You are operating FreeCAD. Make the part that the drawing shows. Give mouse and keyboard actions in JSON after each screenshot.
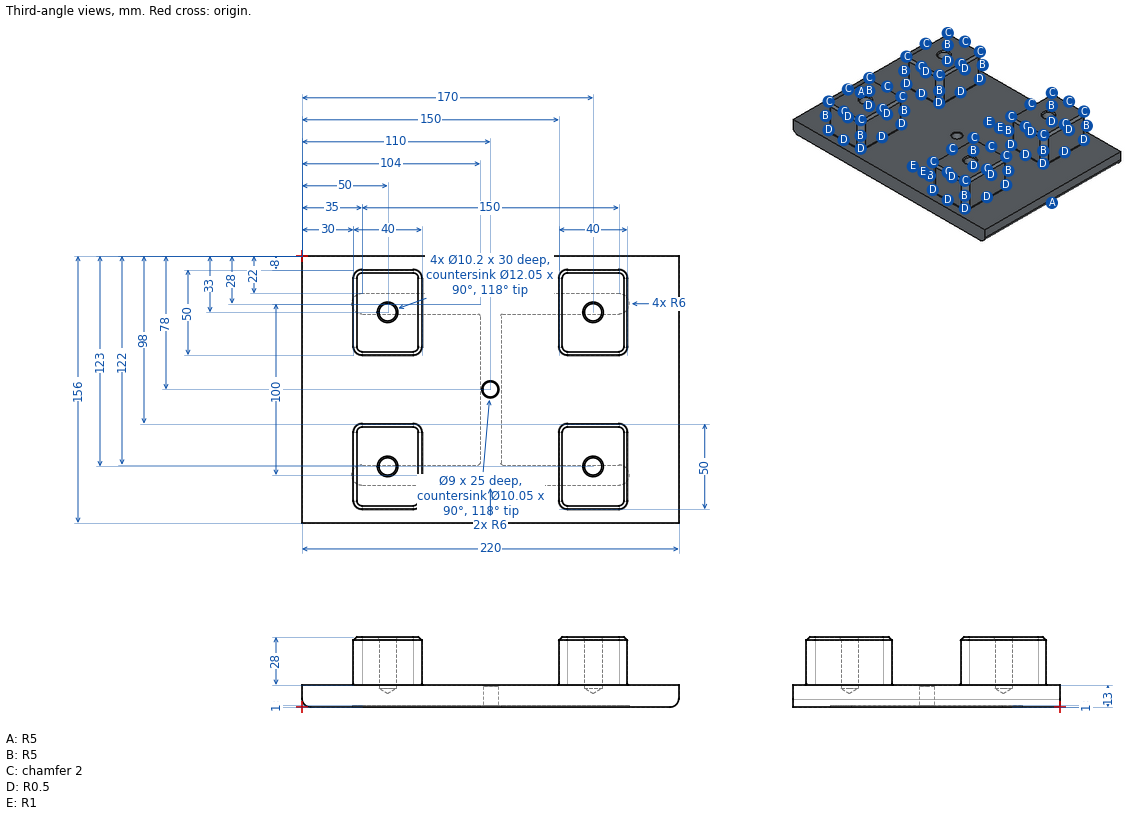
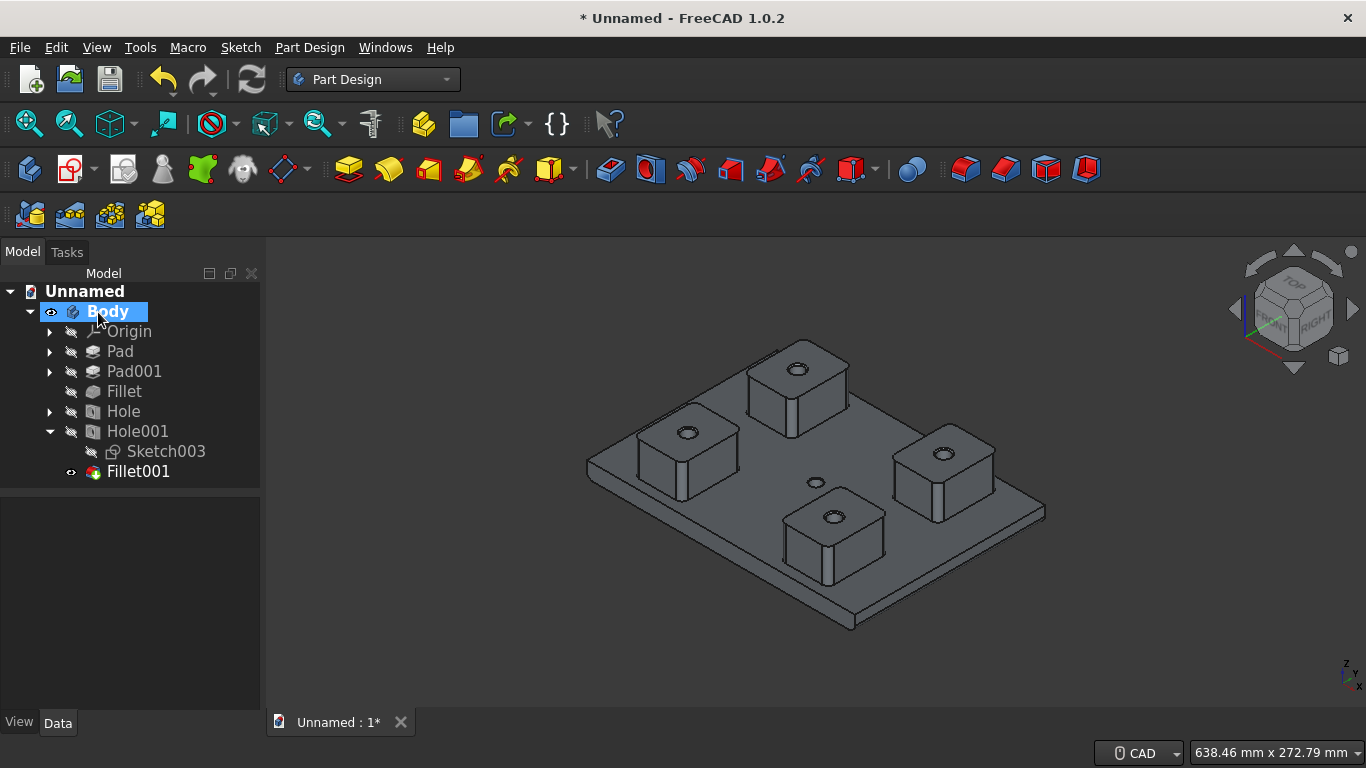
{"action": "left_click", "coordinate": [712, 446]}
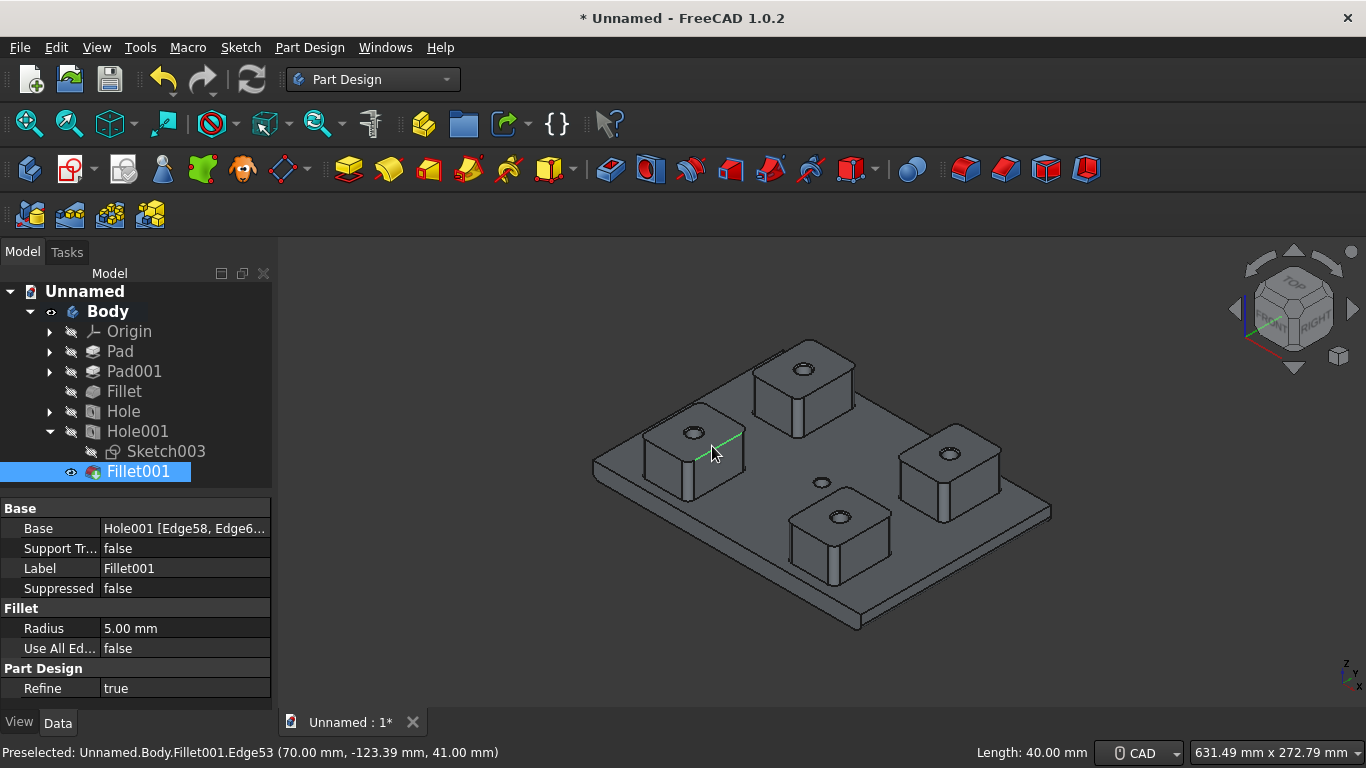
{"action": "left_click", "coordinate": [664, 449], "text": "ctrl"}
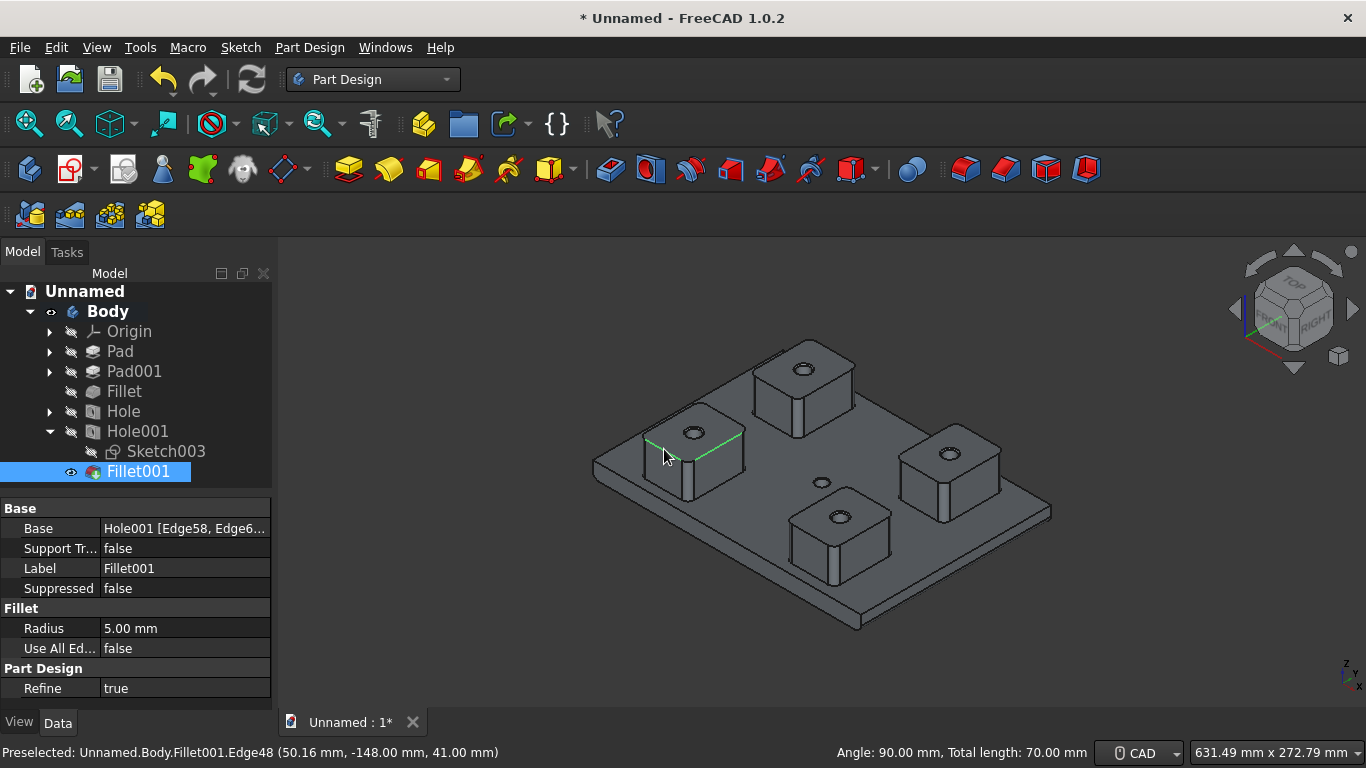
{"action": "left_click", "coordinate": [688, 461], "text": "ctrl"}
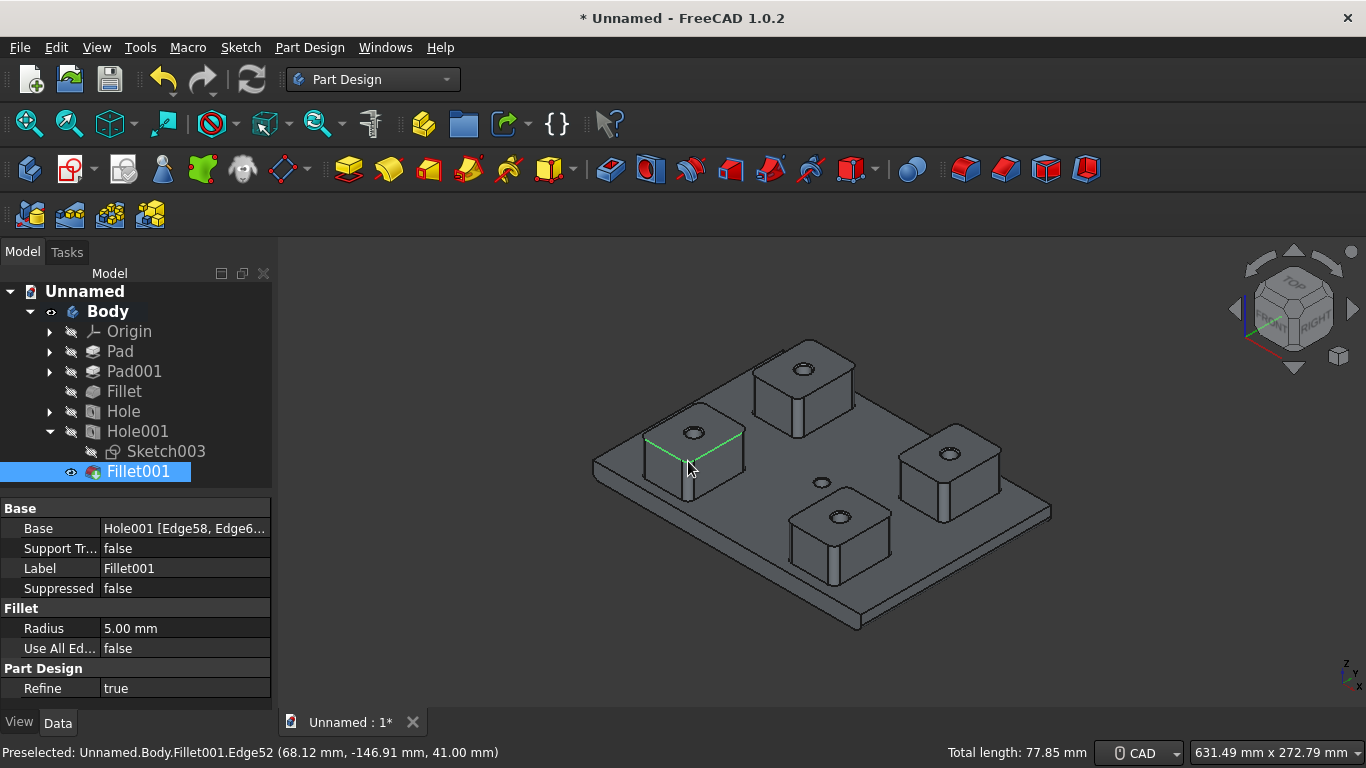
{"action": "left_click", "coordinate": [644, 432], "text": "ctrl"}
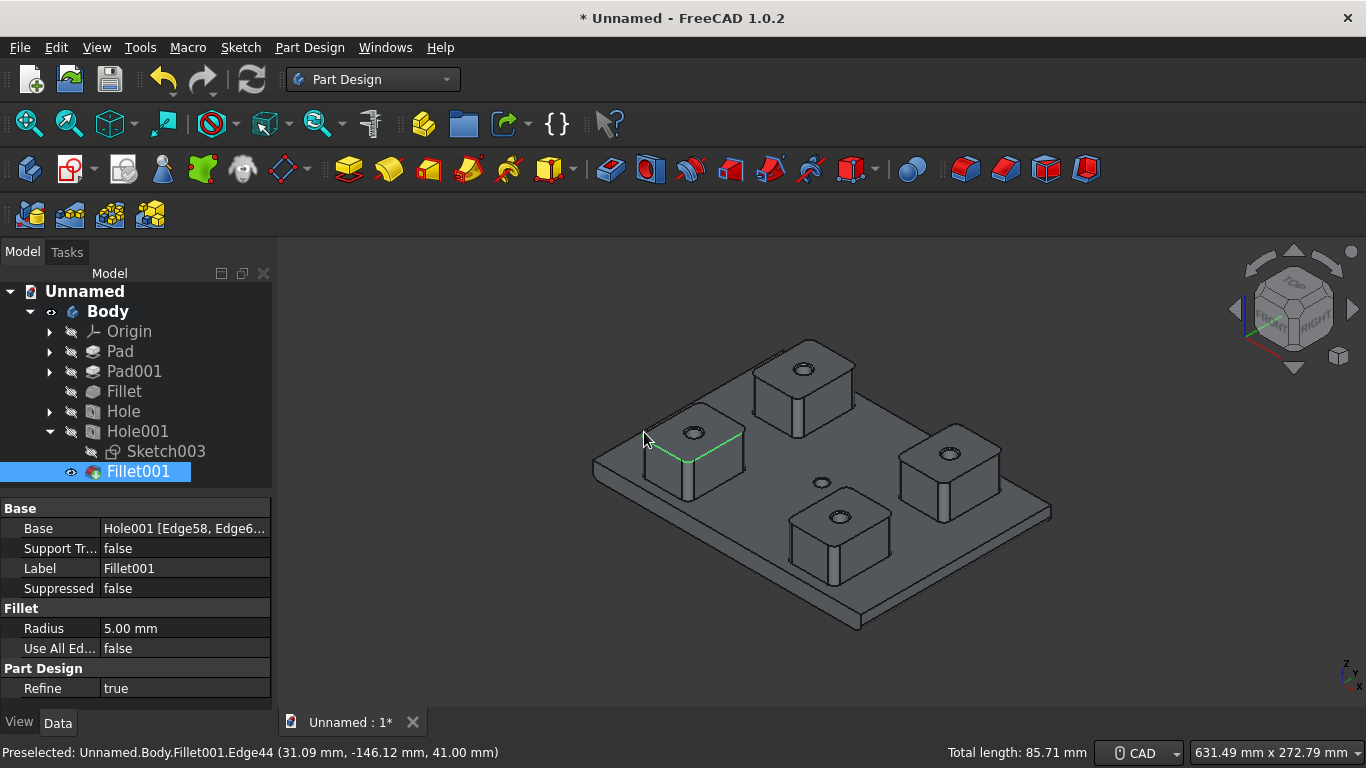
{"action": "left_click", "coordinate": [744, 425], "text": "ctrl"}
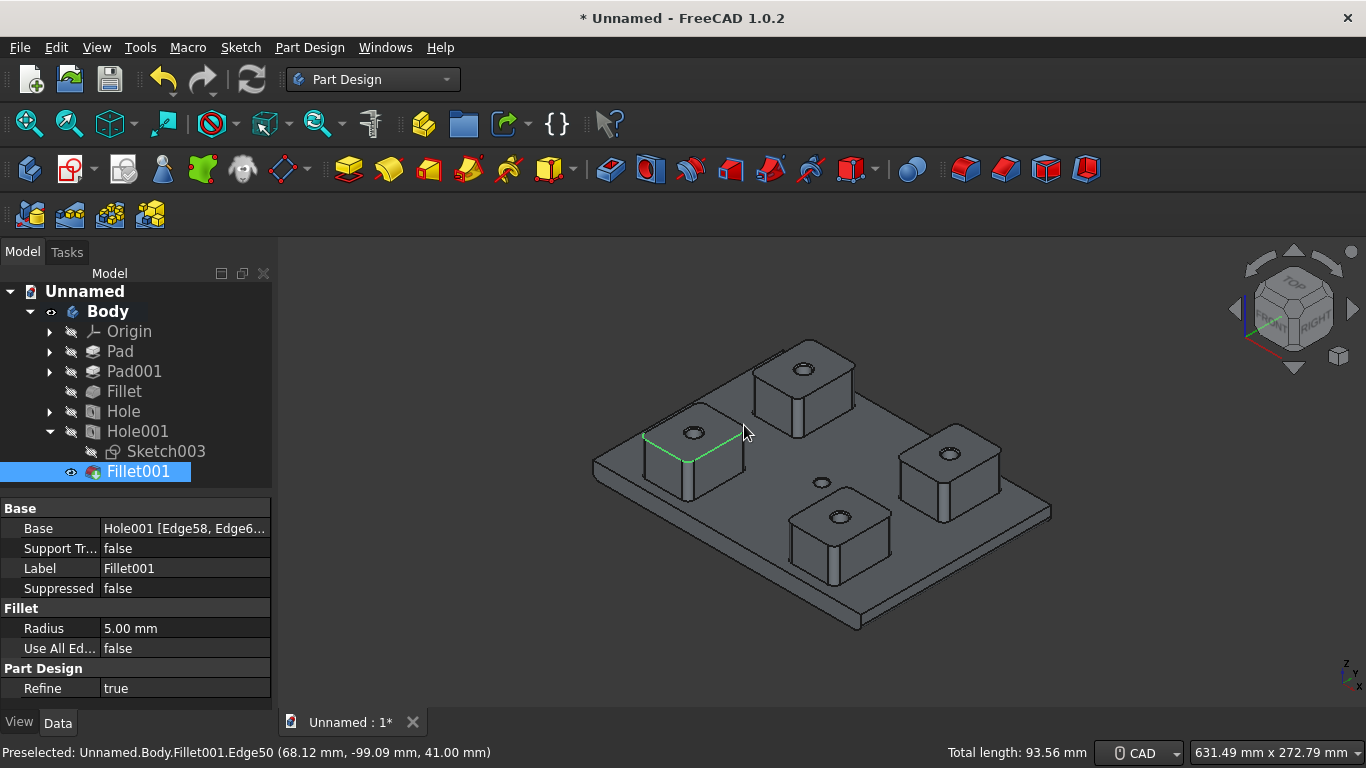
{"action": "left_click", "coordinate": [810, 534], "text": "ctrl"}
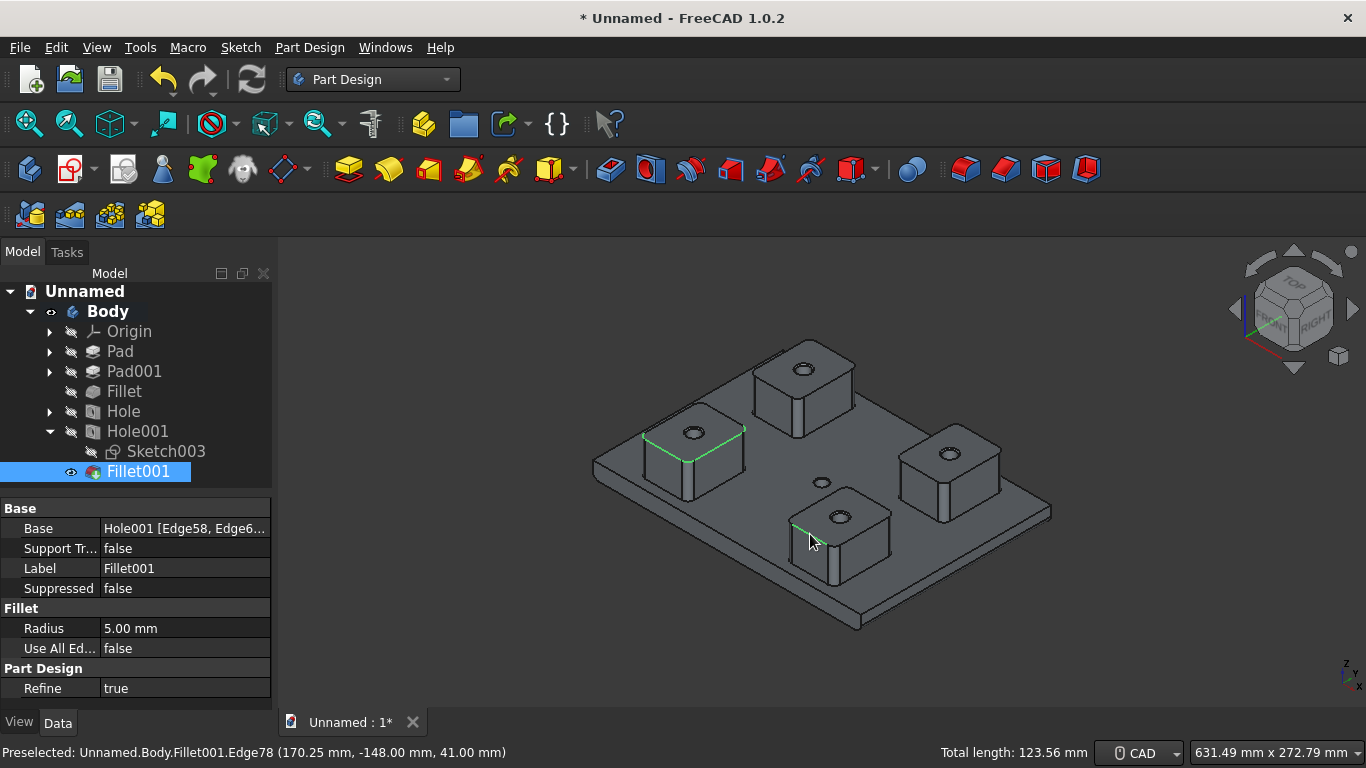
{"action": "left_click", "coordinate": [865, 530], "text": "ctrl"}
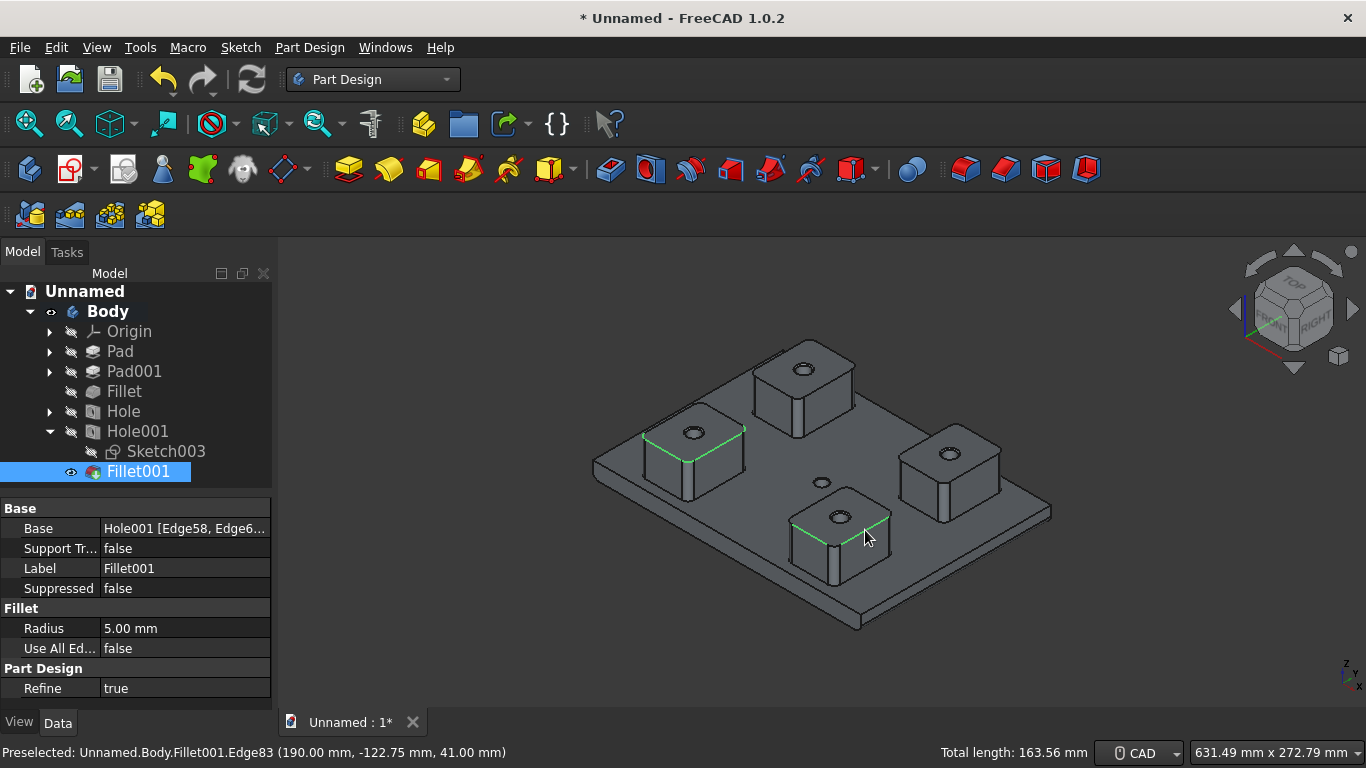
{"action": "left_click", "coordinate": [891, 510], "text": "ctrl"}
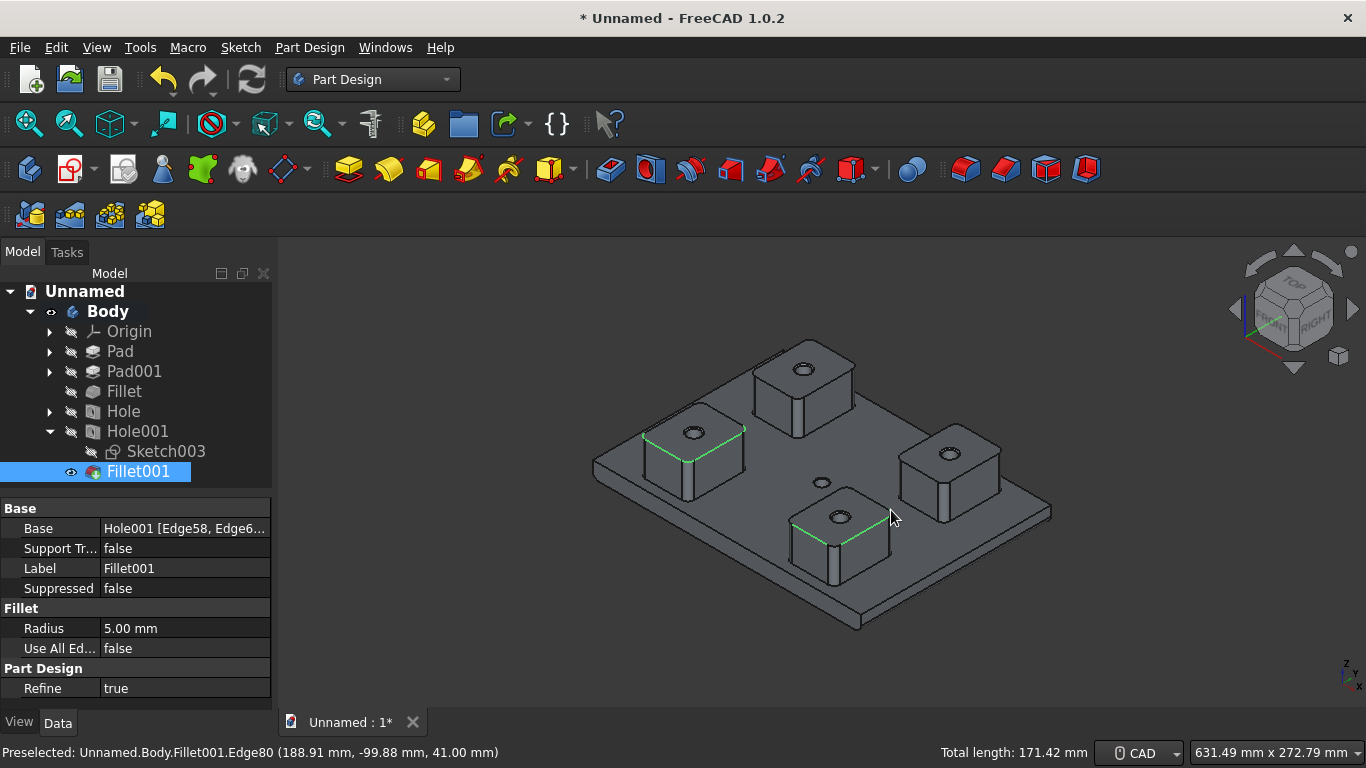
{"action": "left_click", "coordinate": [834, 546], "text": "ctrl"}